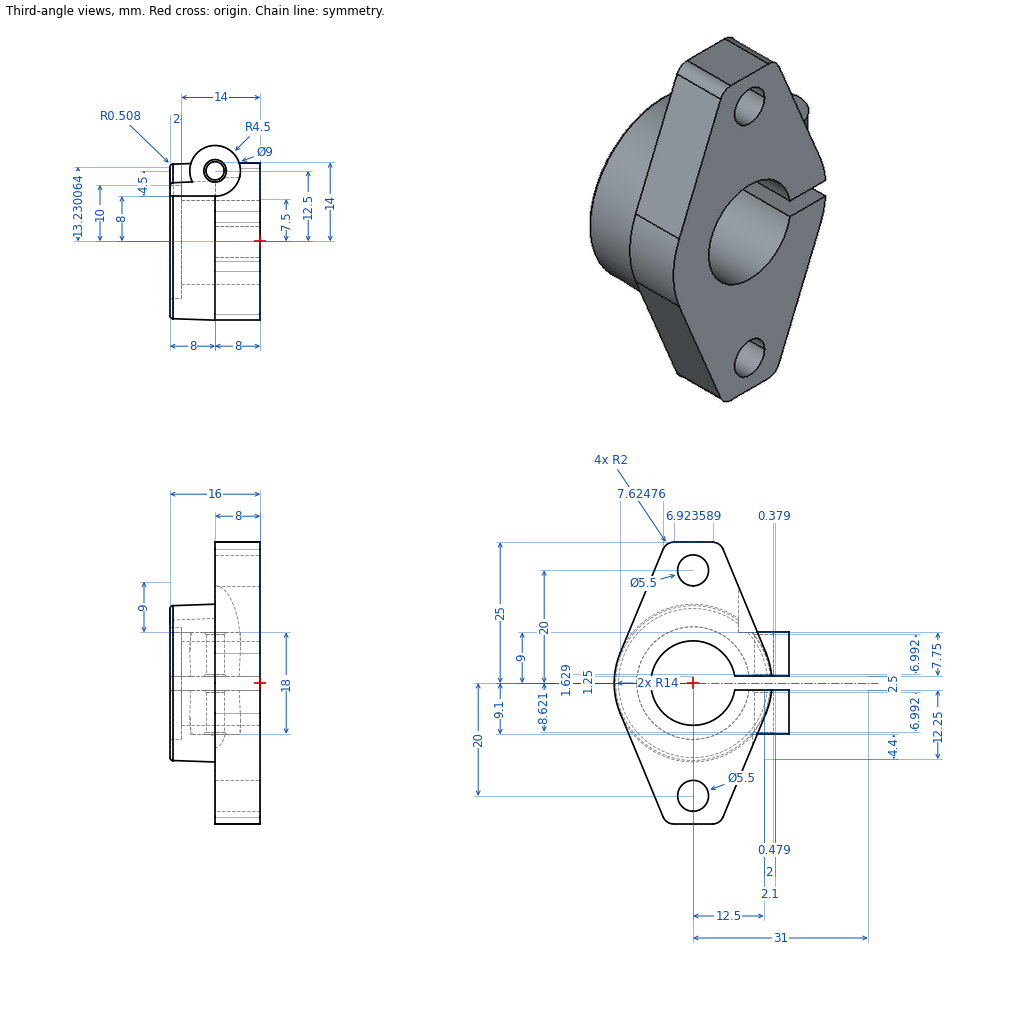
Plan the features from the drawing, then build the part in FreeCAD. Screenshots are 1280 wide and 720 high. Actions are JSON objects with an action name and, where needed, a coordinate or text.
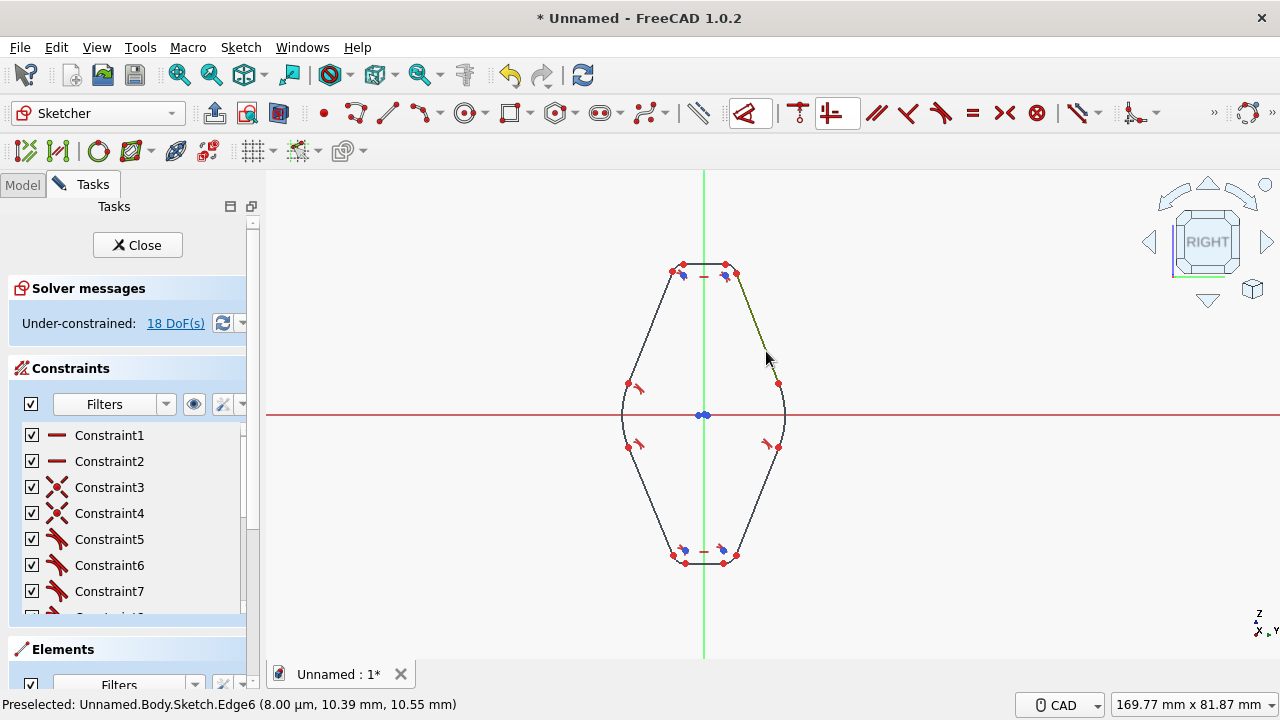
{"action": "left_click", "coordinate": [784, 429]}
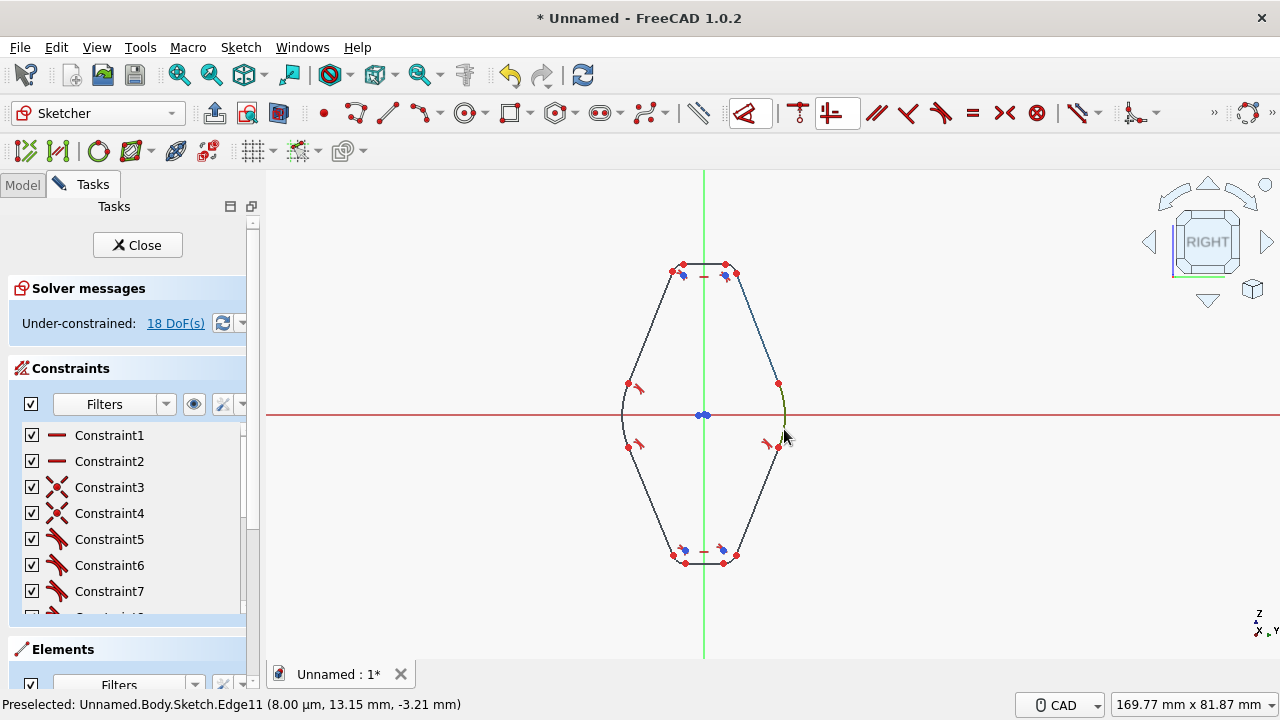
{"action": "left_click", "coordinate": [942, 114]}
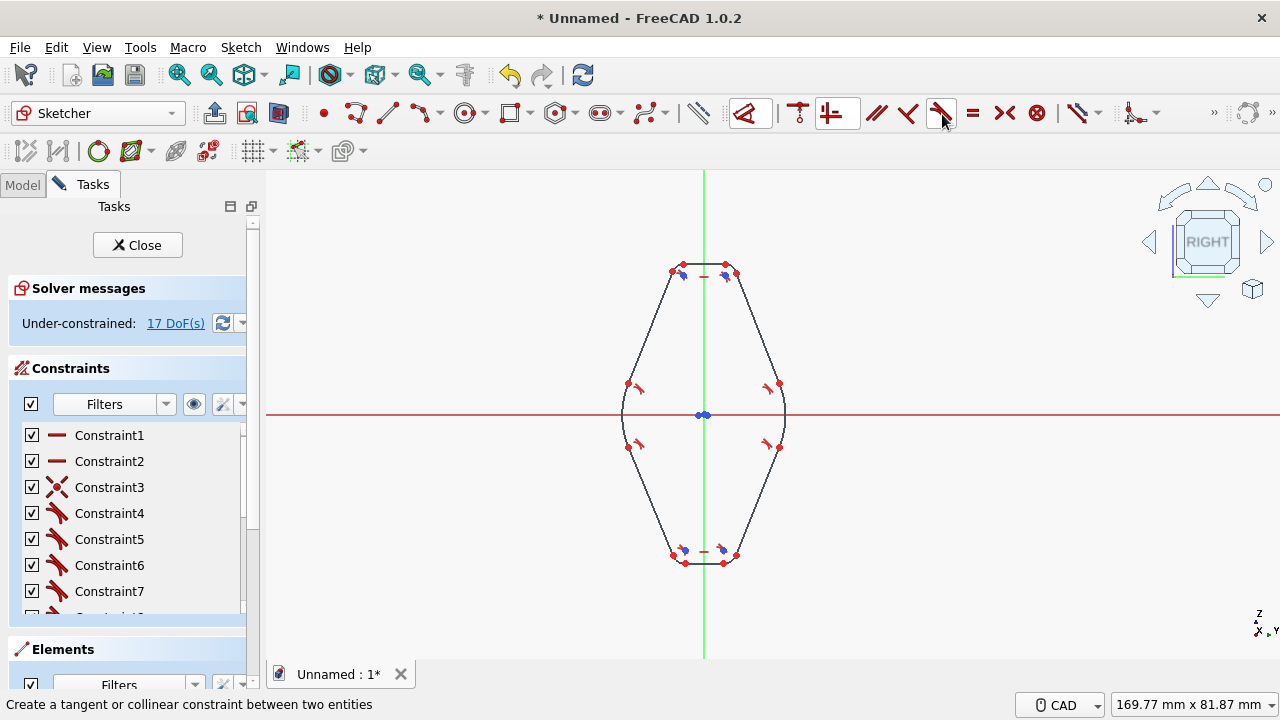
{"action": "left_click", "coordinate": [767, 351]}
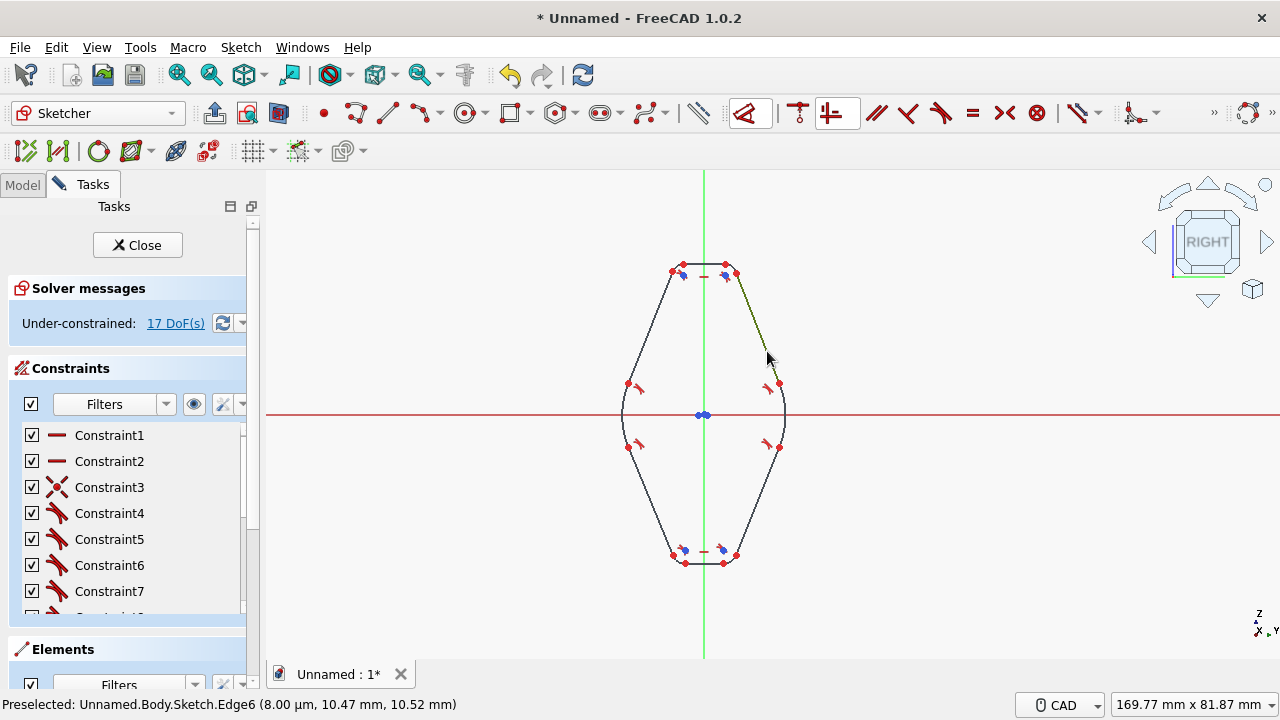
{"action": "scroll", "coordinate": [733, 267], "scroll_direction": "up", "scroll_amount": 3}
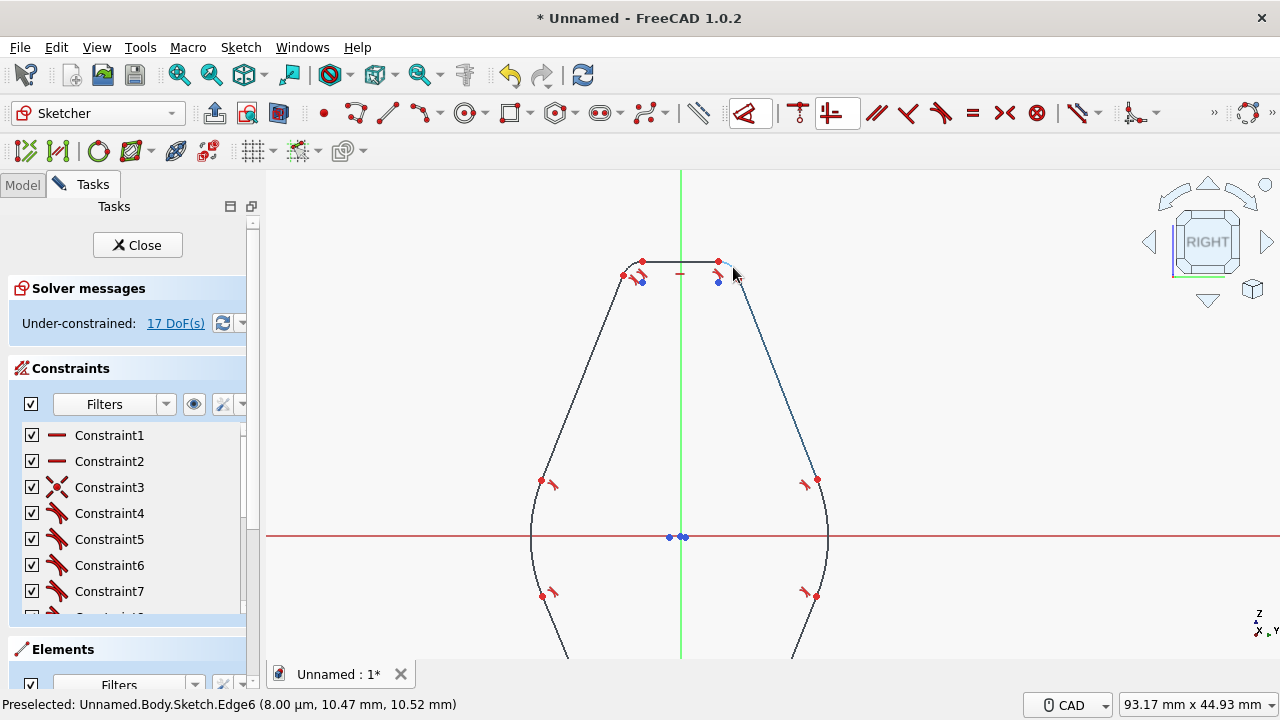
{"action": "left_click", "coordinate": [732, 267]}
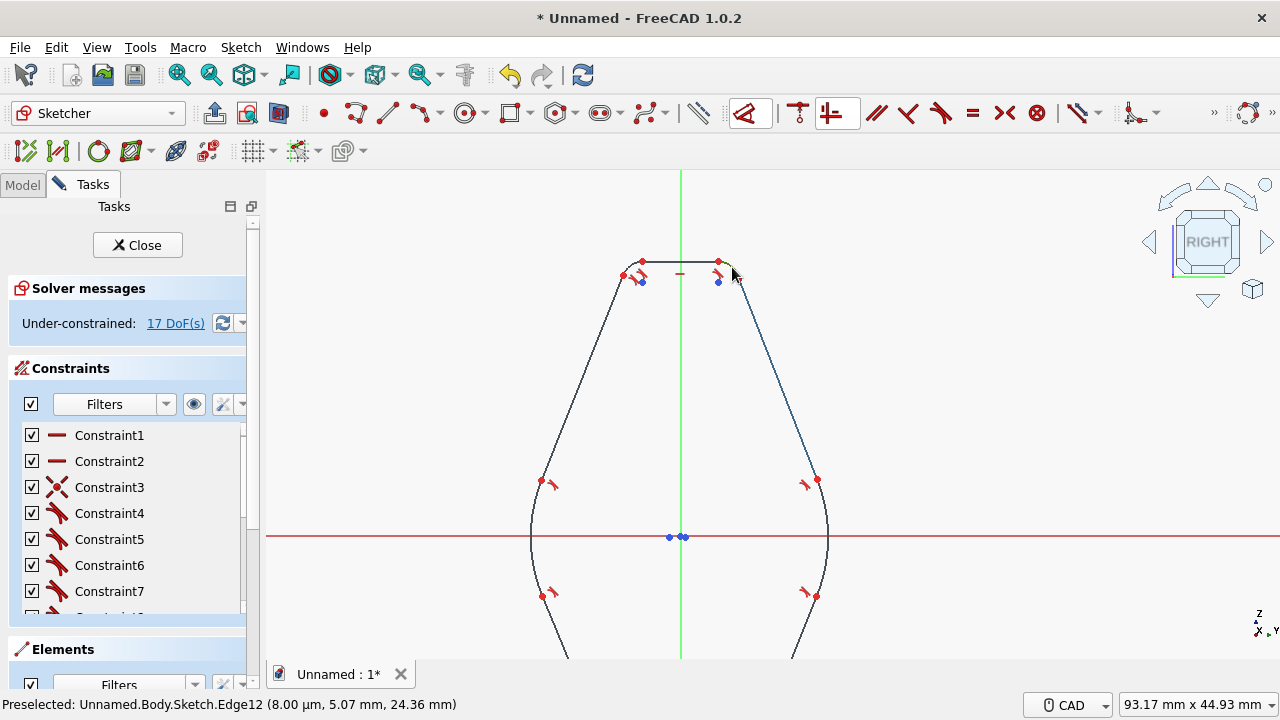
{"action": "left_click", "coordinate": [942, 114]}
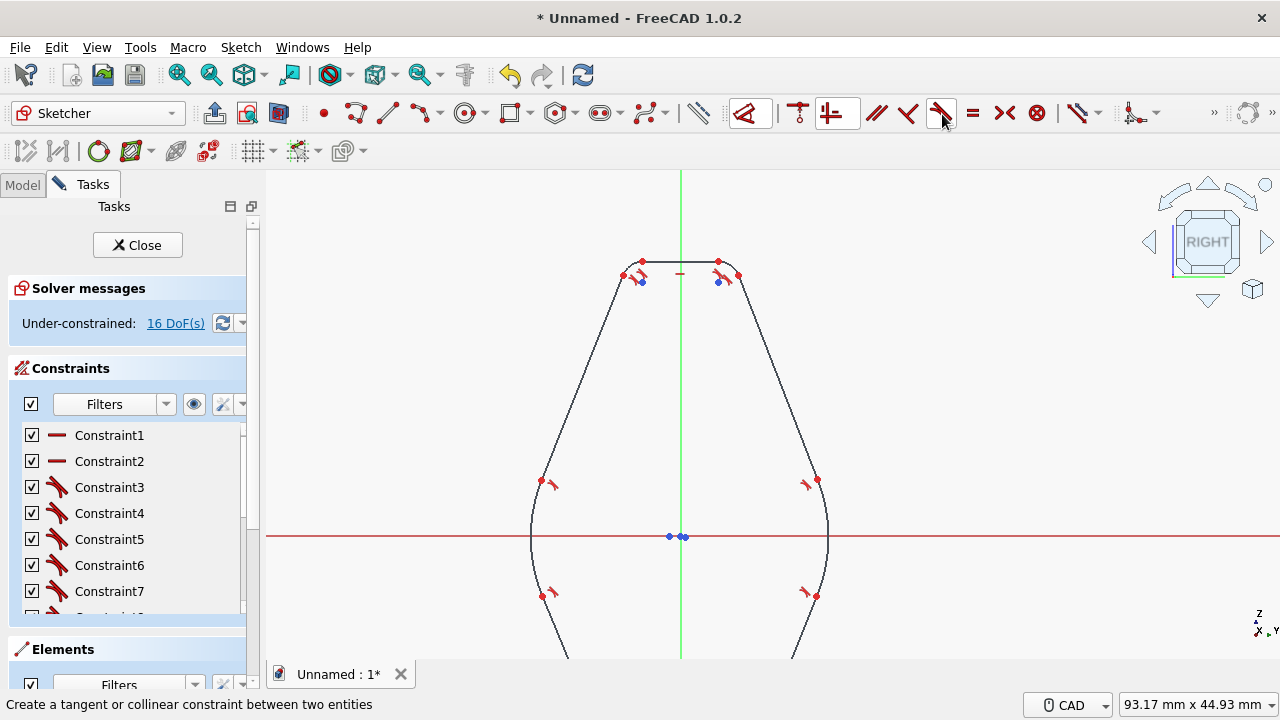
{"action": "left_click", "coordinate": [532, 514]}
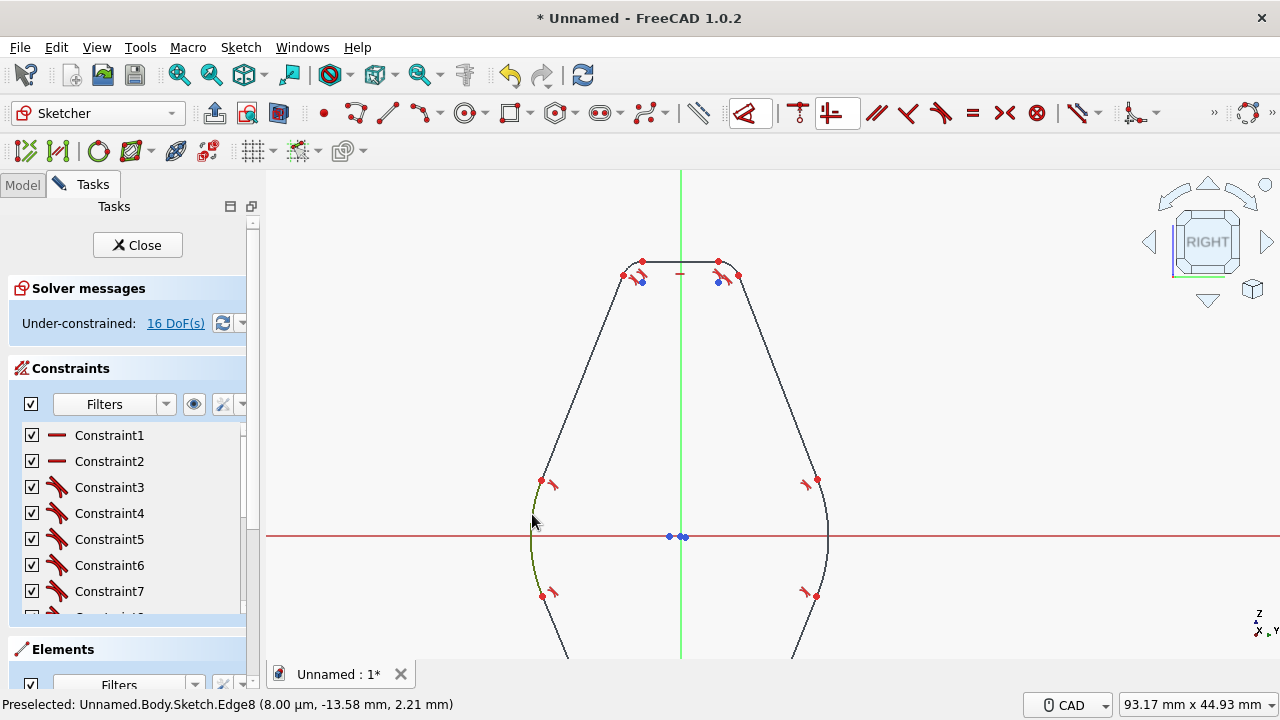
{"action": "left_click", "coordinate": [826, 562]}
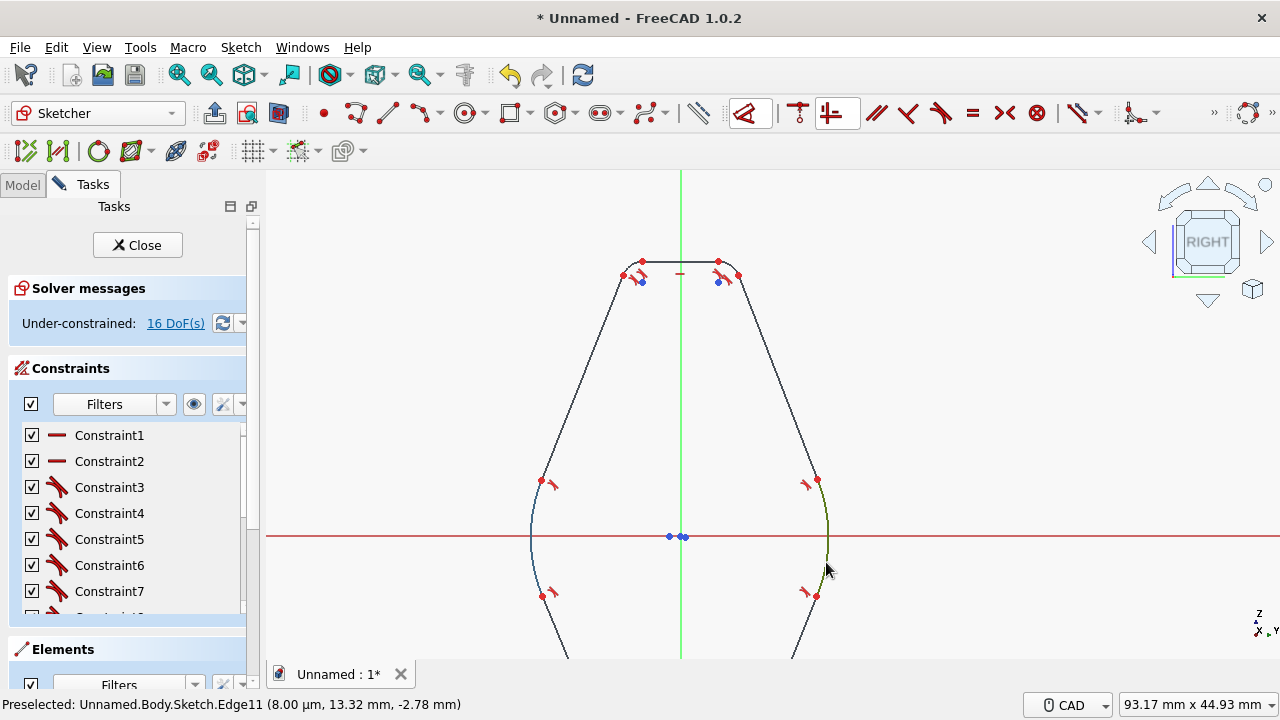
{"action": "left_click", "coordinate": [798, 114]}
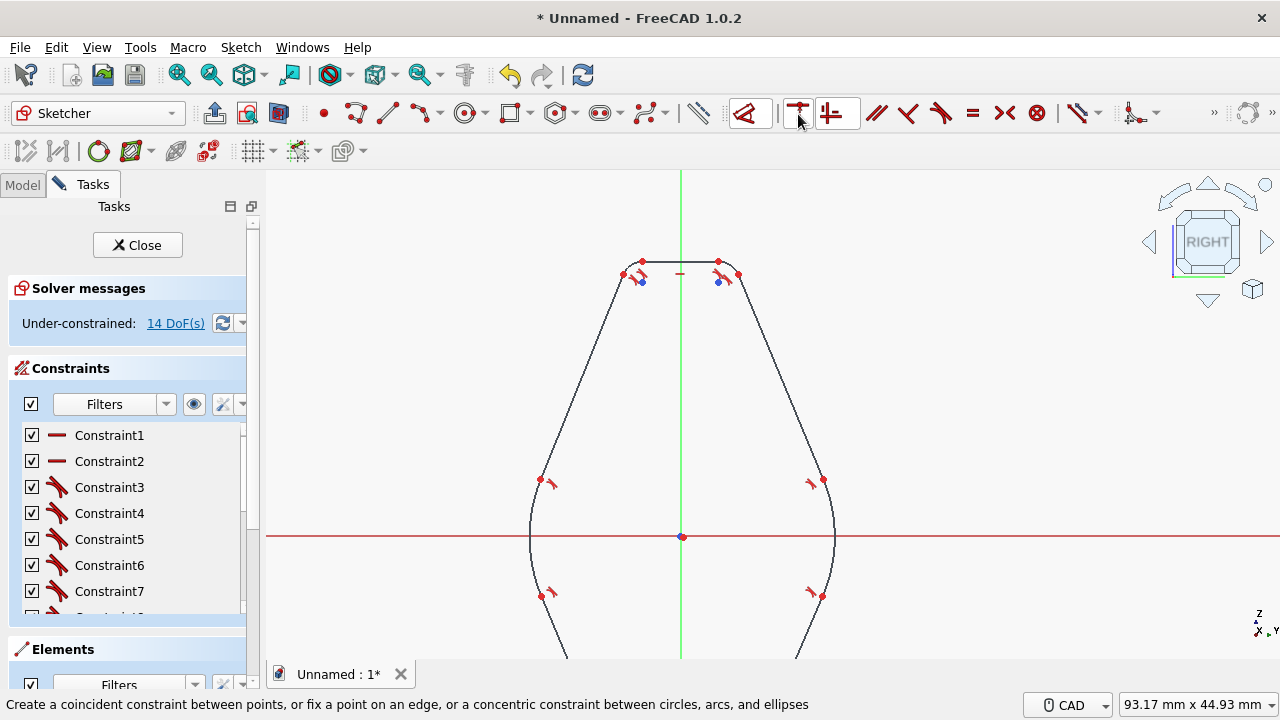
{"action": "scroll", "coordinate": [682, 537], "scroll_direction": "up", "scroll_amount": 4}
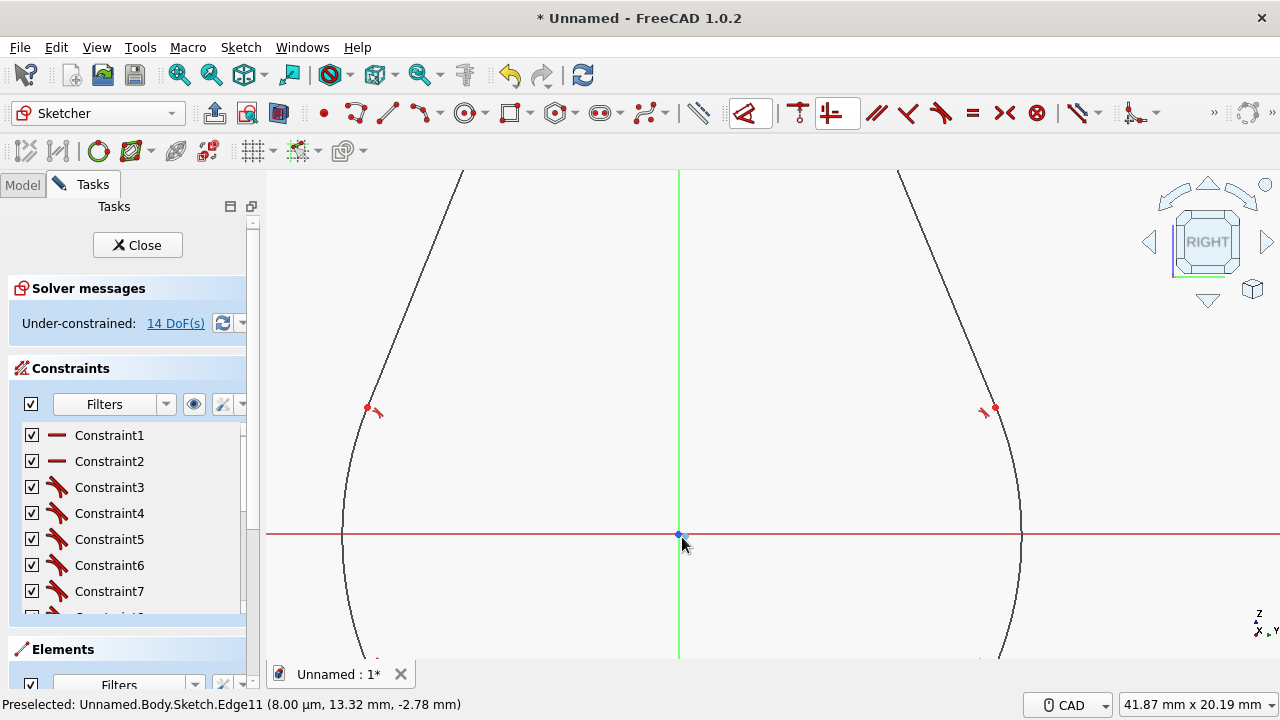
{"action": "left_click_drag", "start_coordinate": [669, 524], "coordinate": [695, 546]}